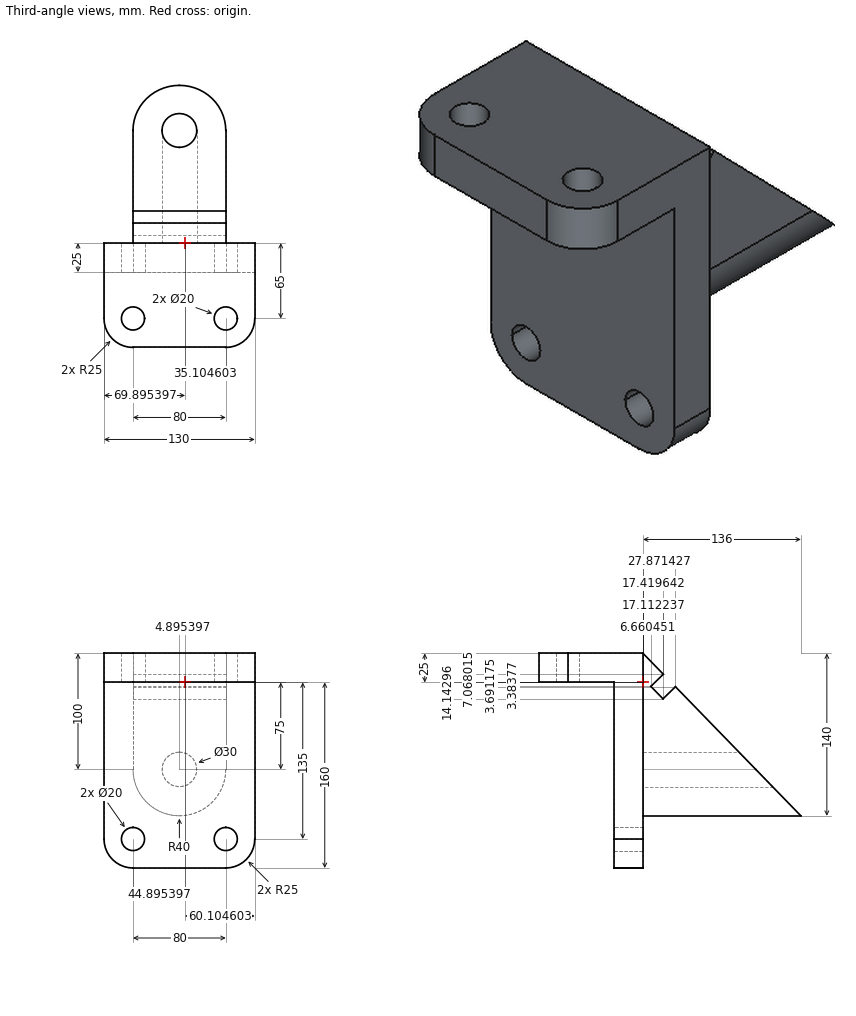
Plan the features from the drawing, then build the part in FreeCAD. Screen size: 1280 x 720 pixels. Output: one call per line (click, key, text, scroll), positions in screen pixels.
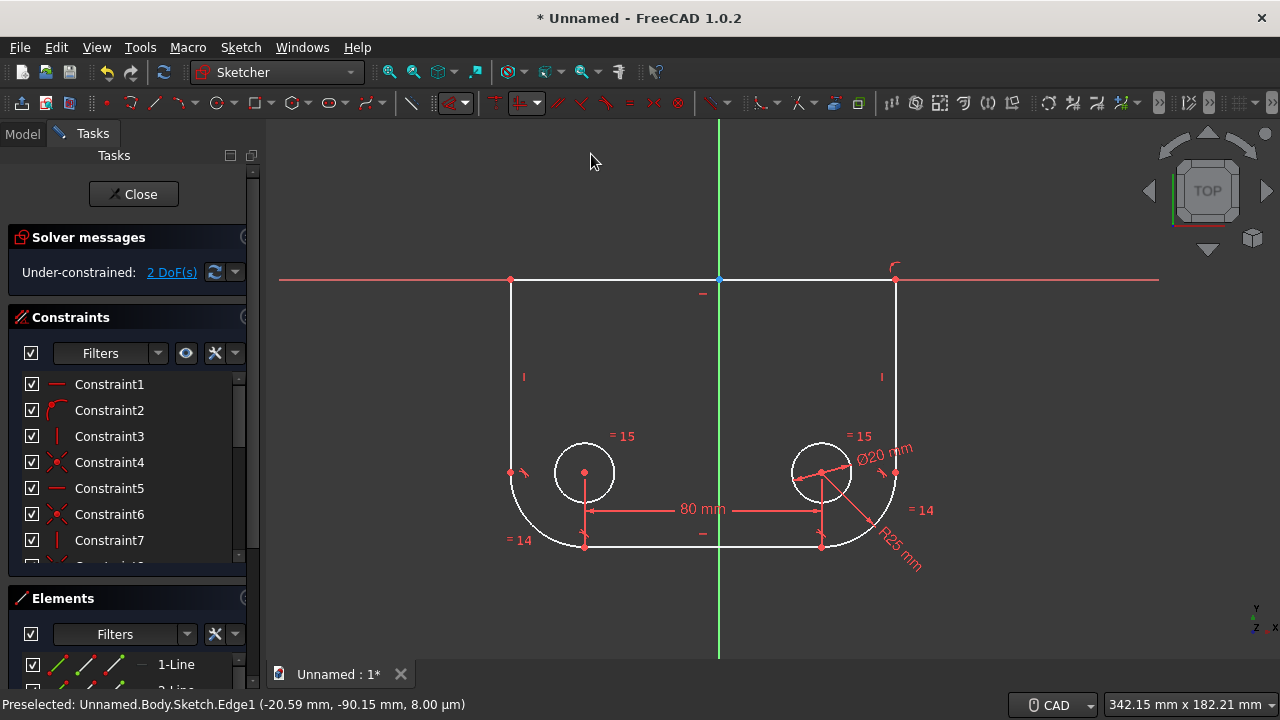
click(896, 415)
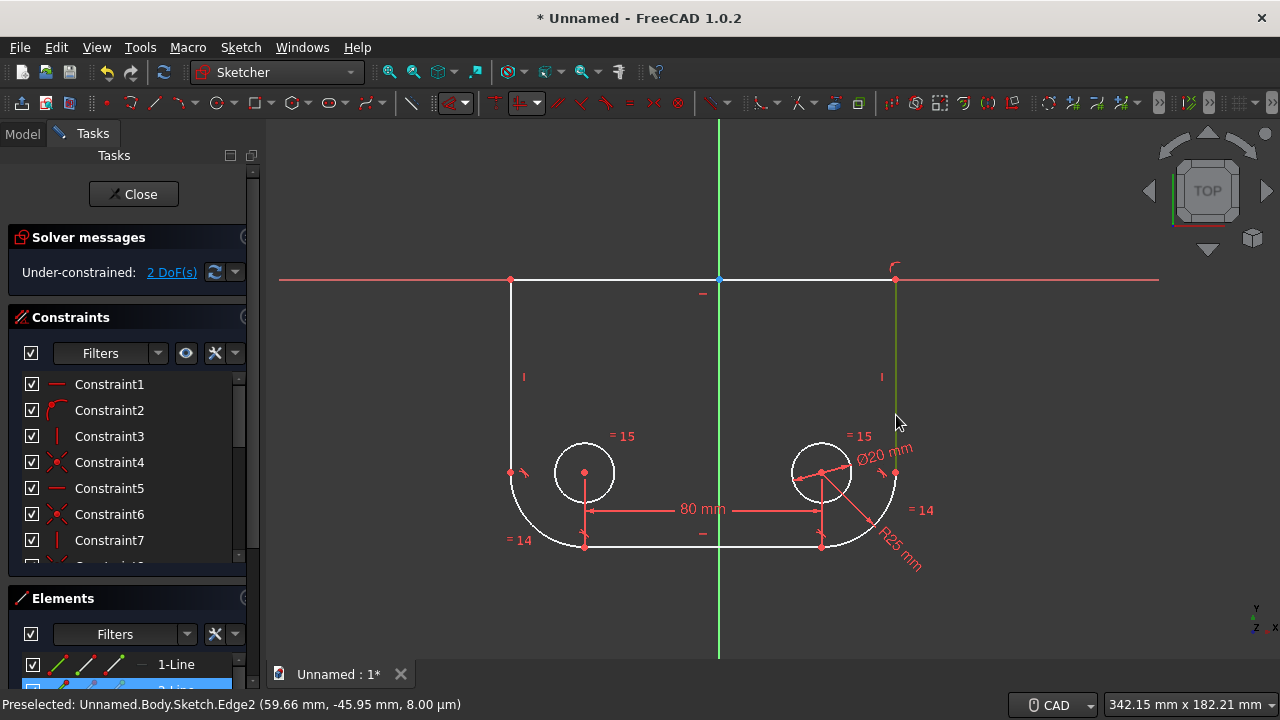
key(i)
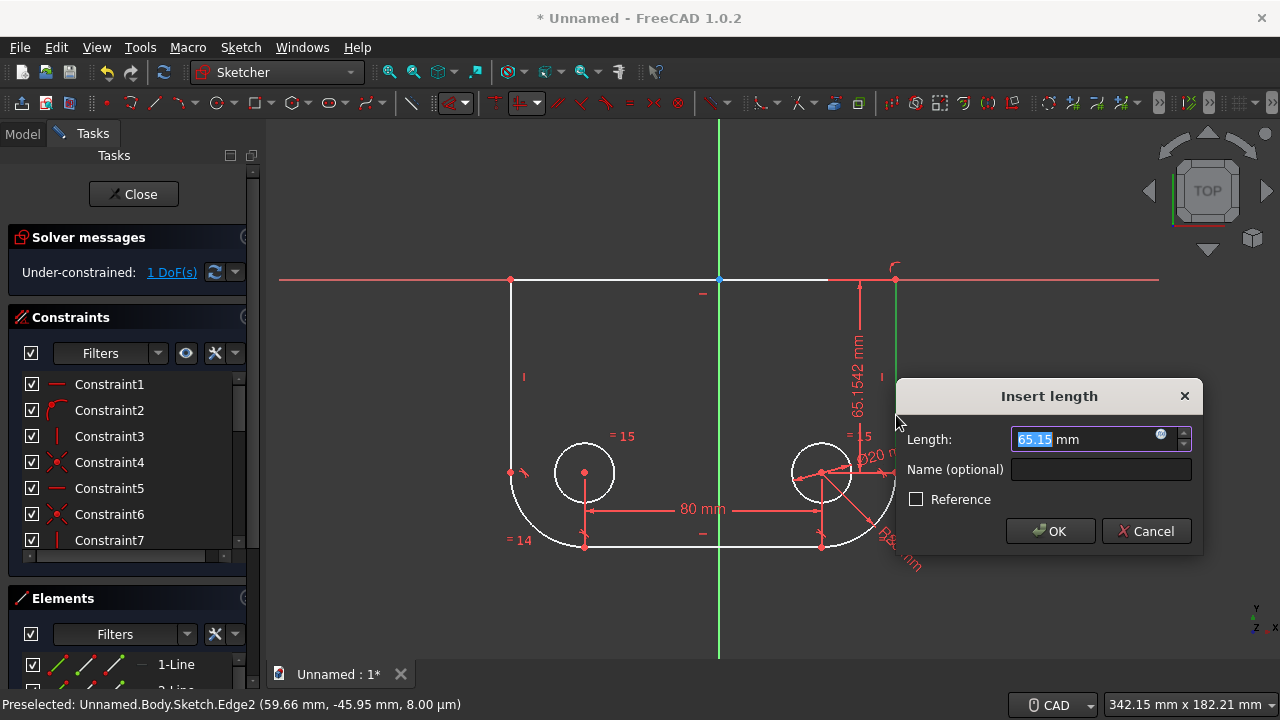
text(65)
key(Return)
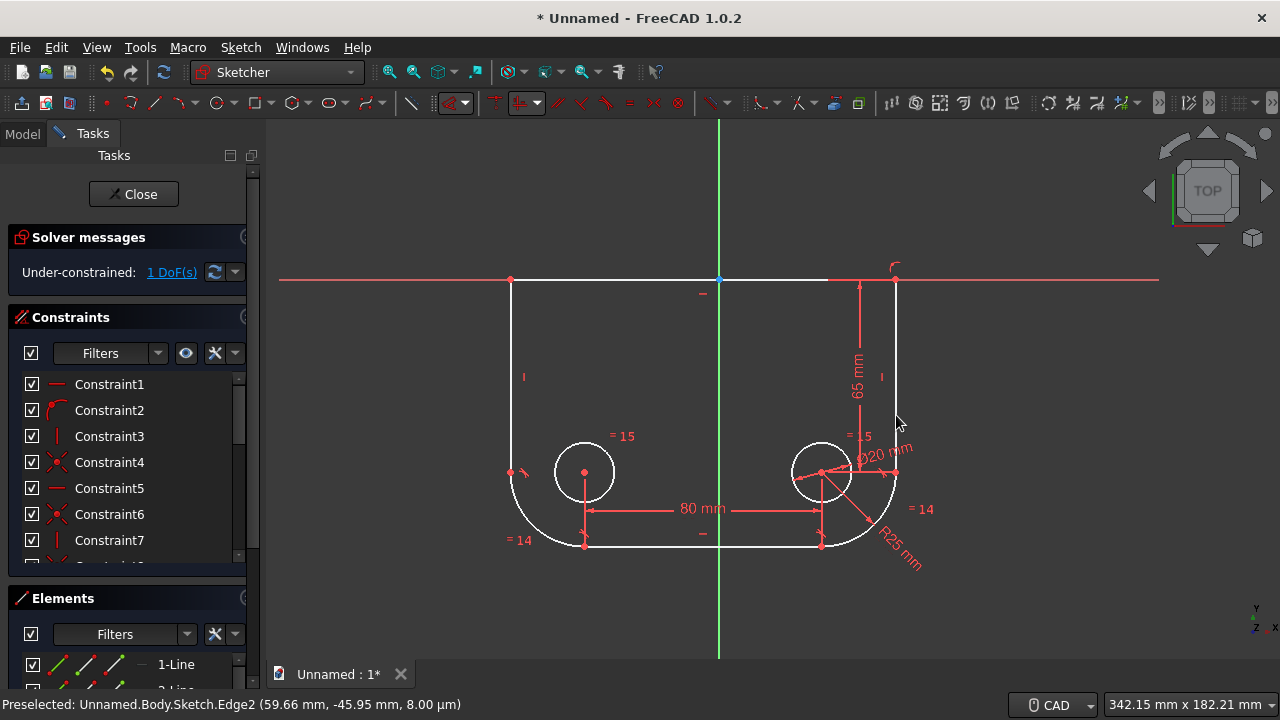
click(822, 472)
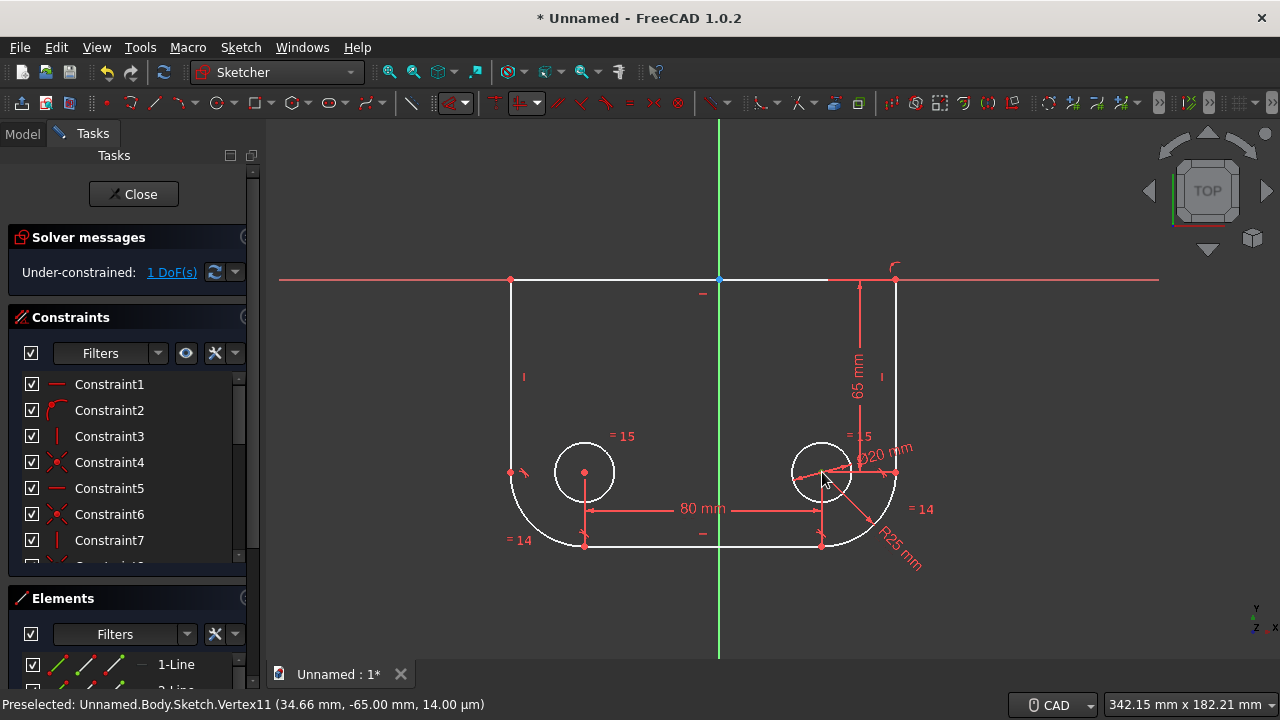
key(l)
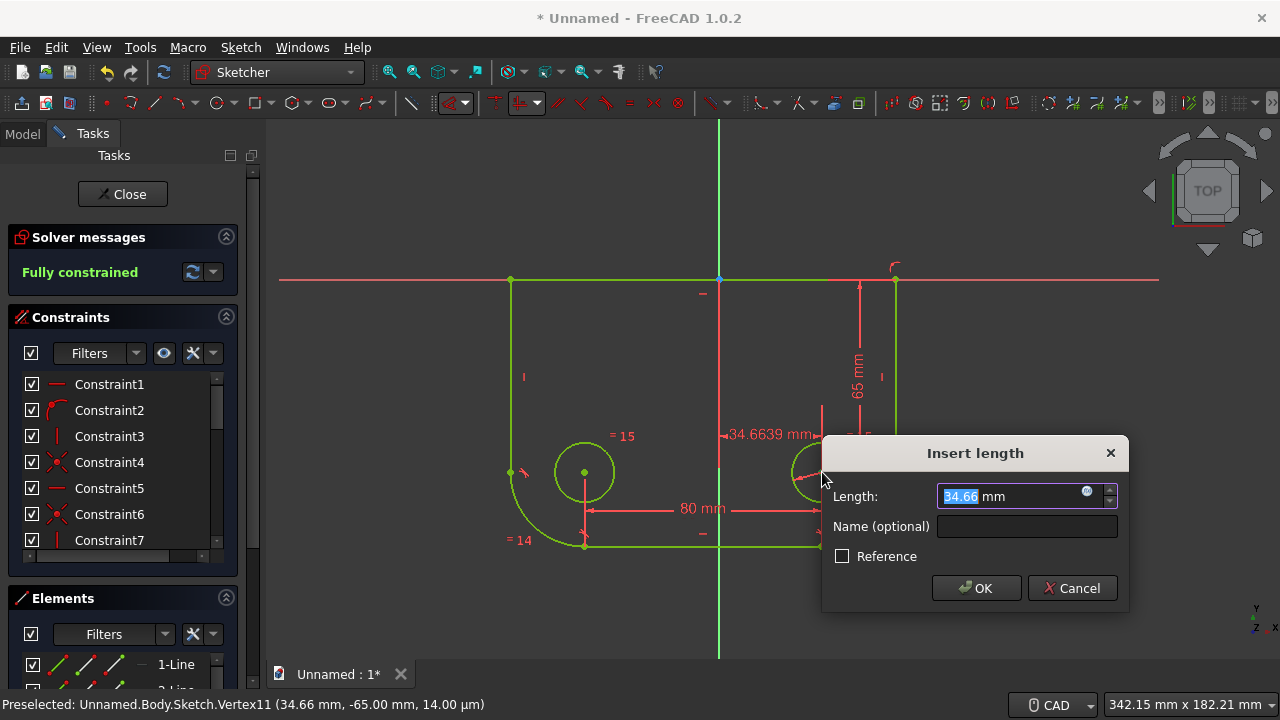
text(35.104603)
key(Return)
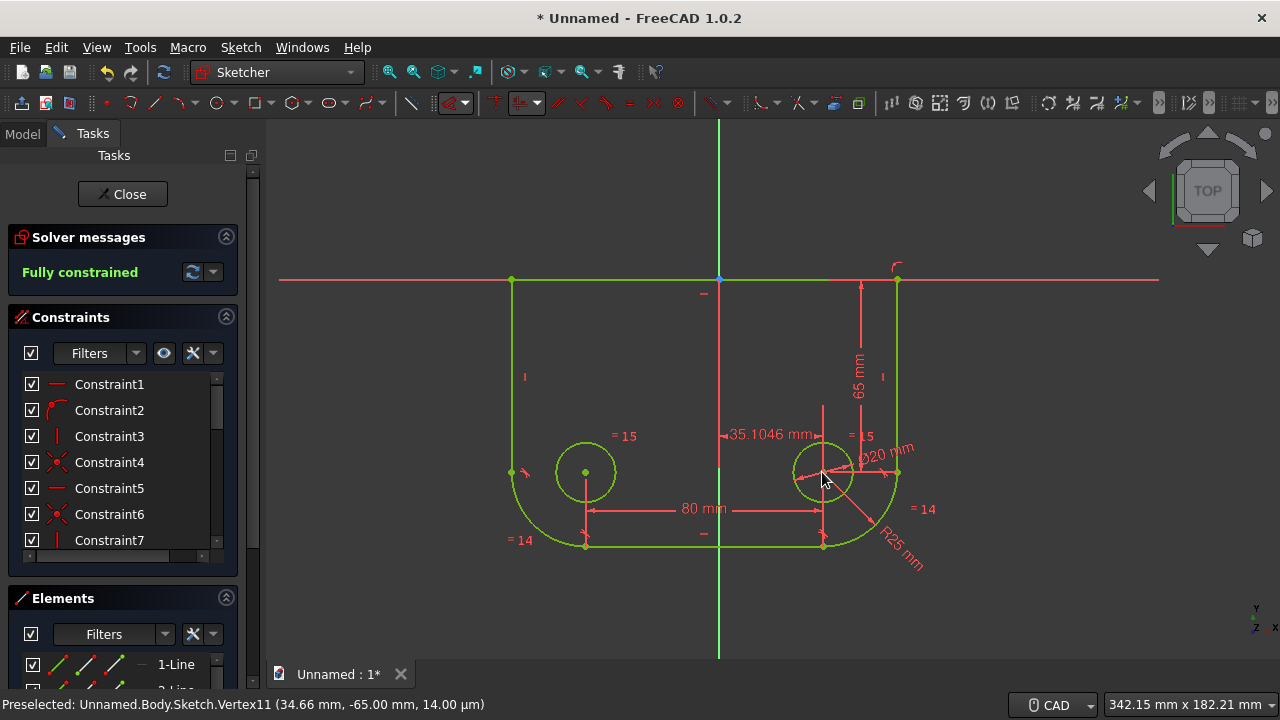
click(123, 194)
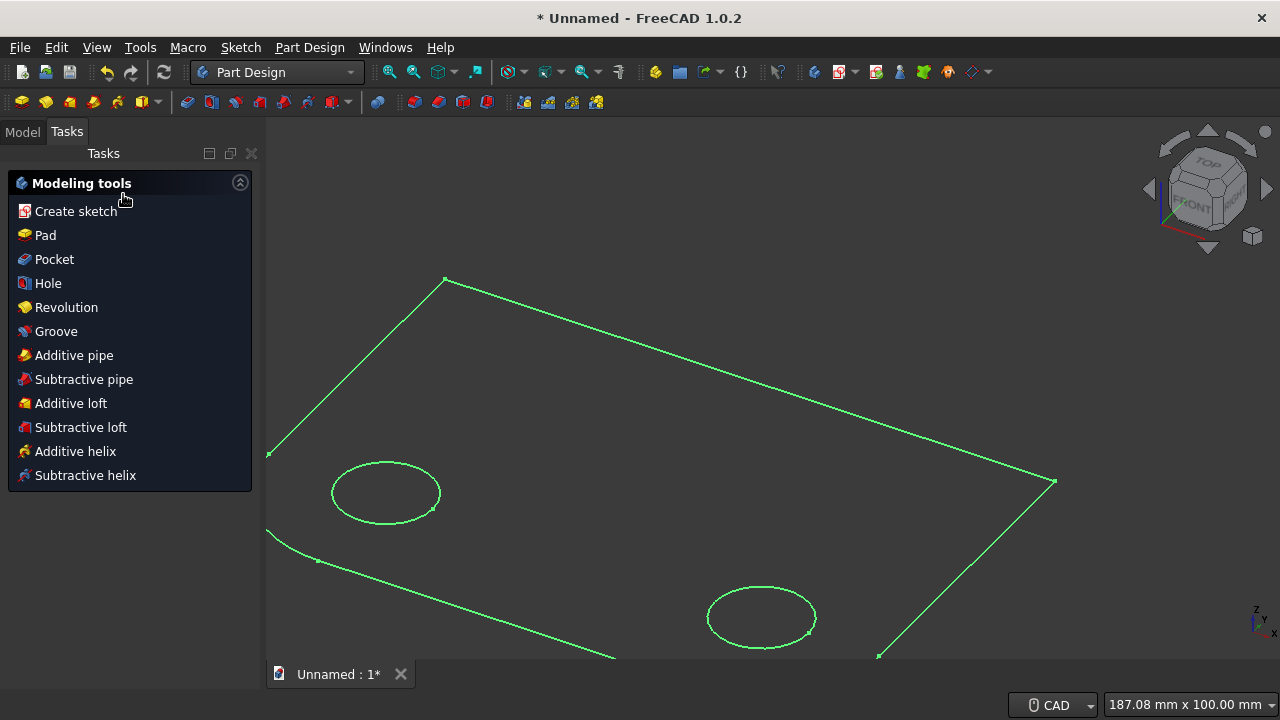
click(22, 102)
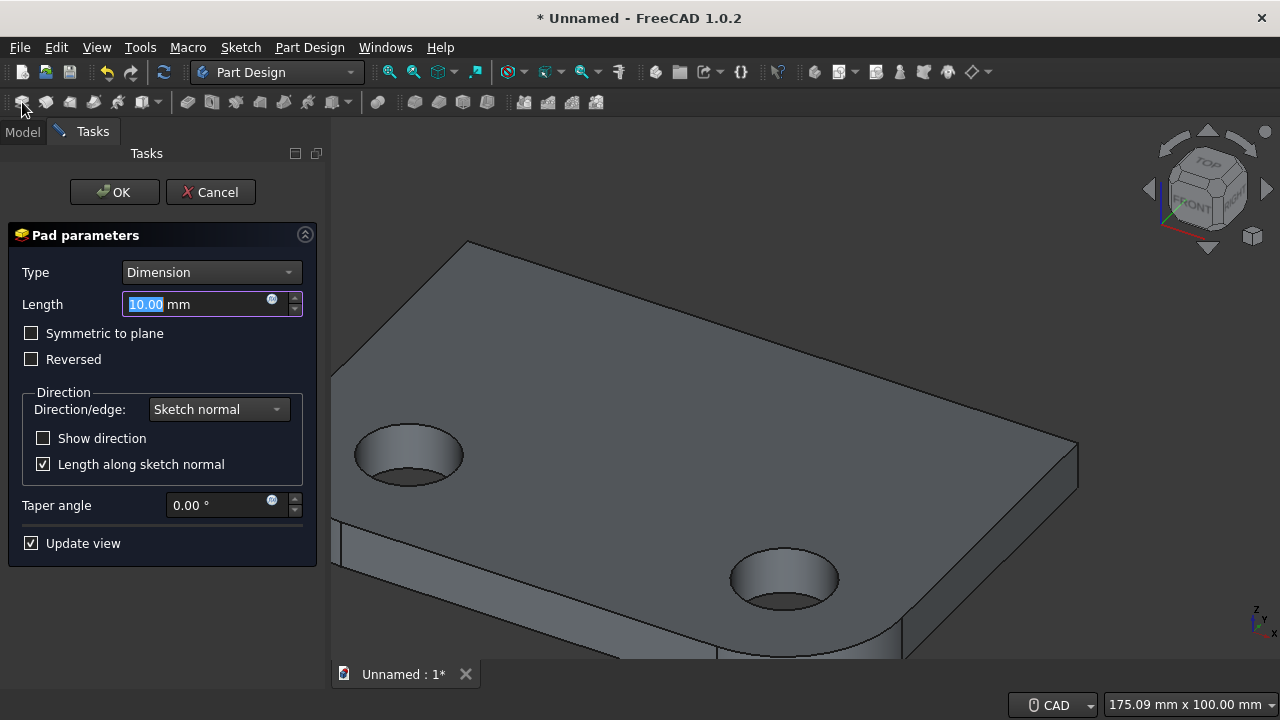
text(25)
key(Tab)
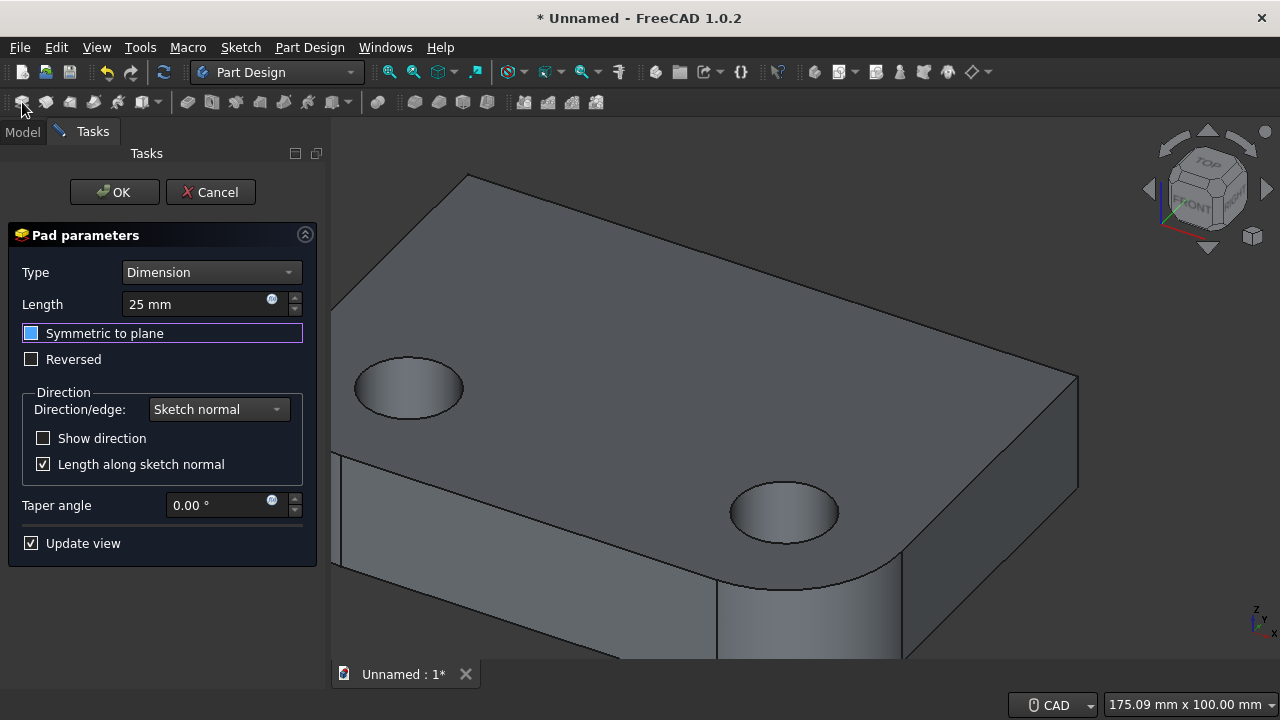
click(115, 192)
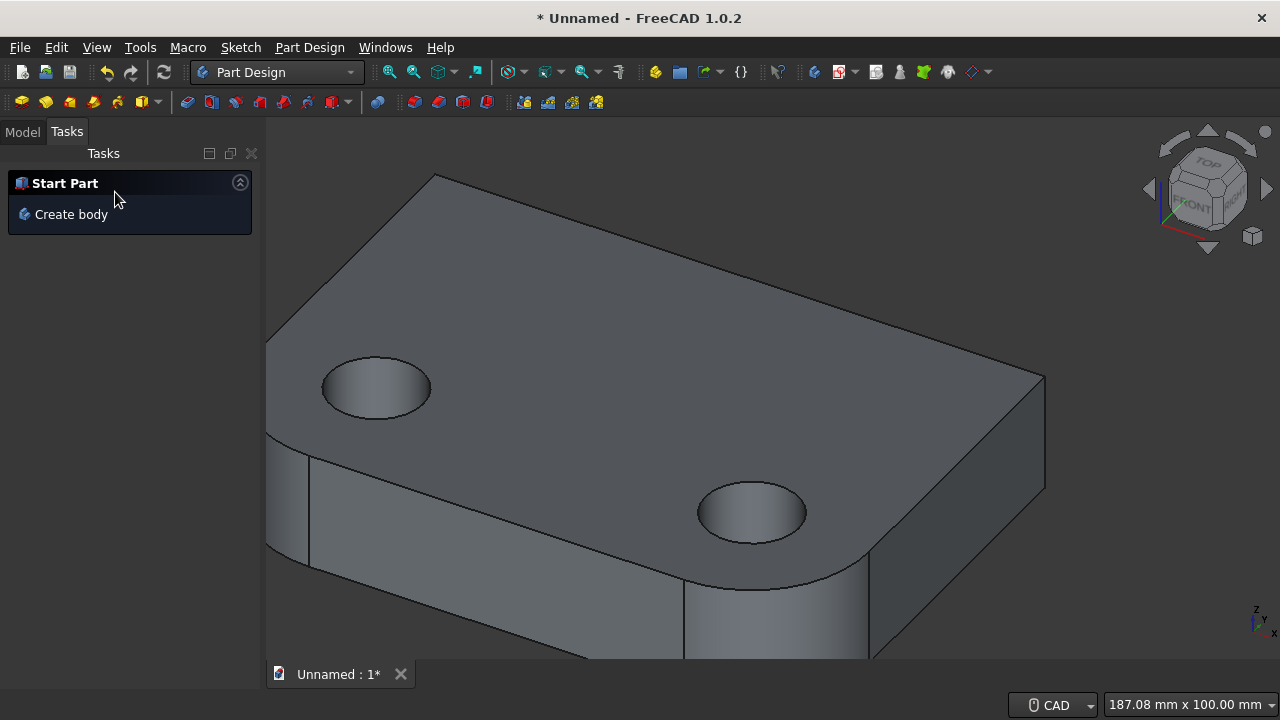
click(390, 72)